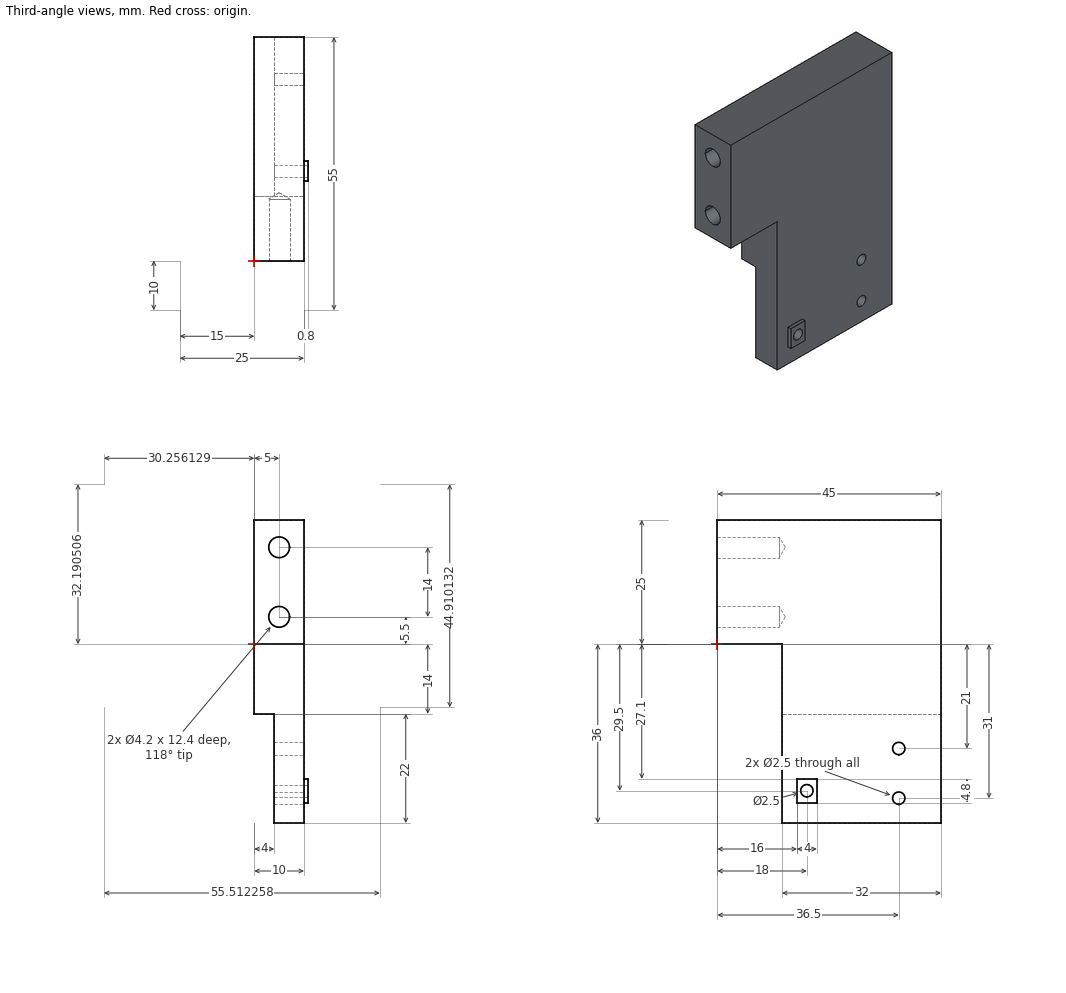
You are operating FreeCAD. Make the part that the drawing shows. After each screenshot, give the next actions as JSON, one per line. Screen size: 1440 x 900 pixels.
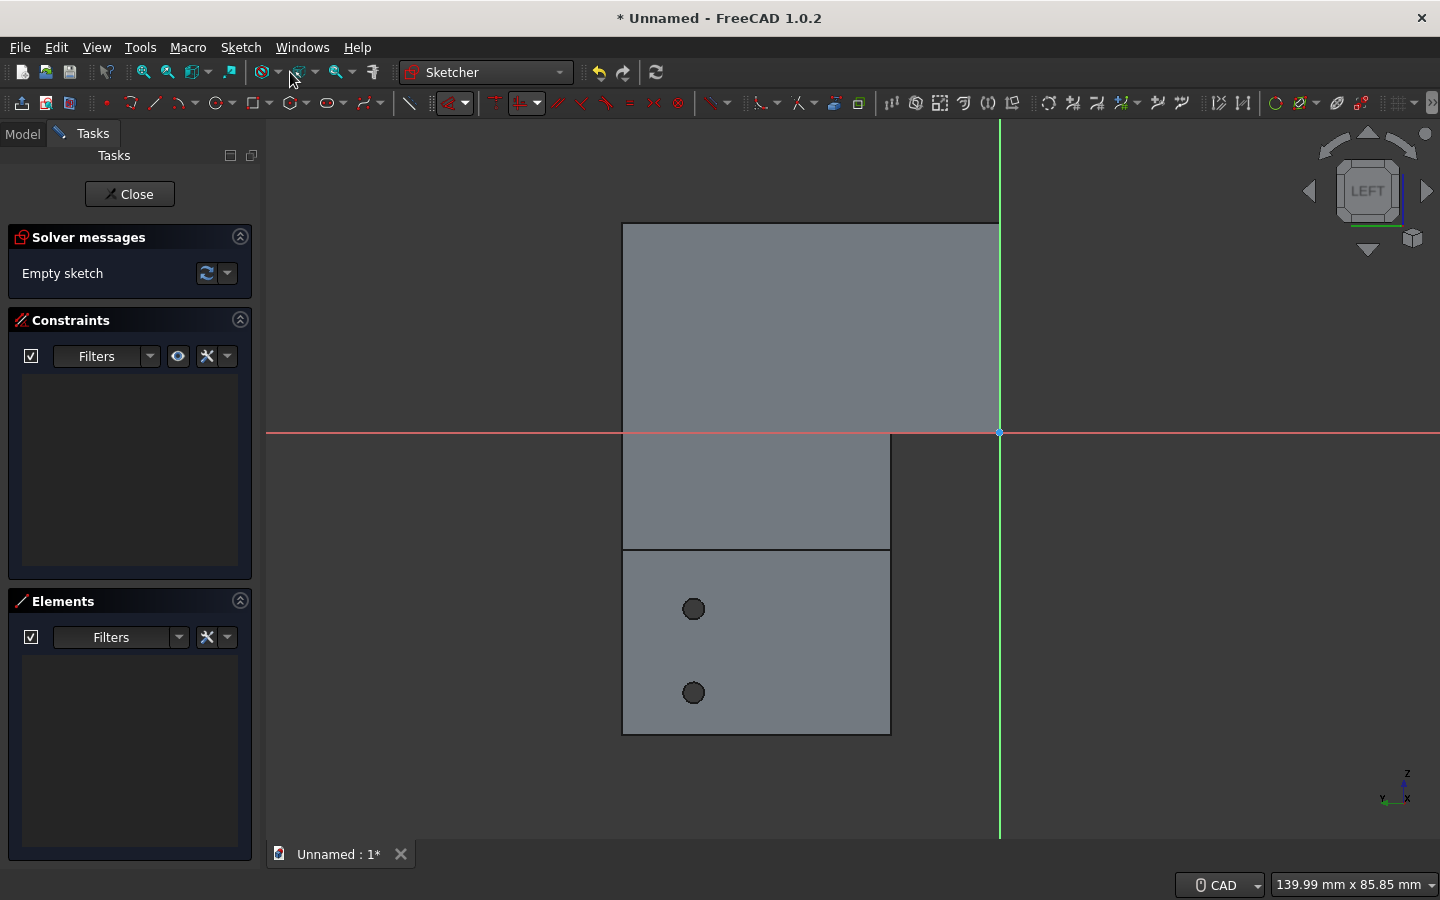
{"action": "scroll", "coordinate": [852, 691], "scroll_direction": "up", "scroll_amount": 15}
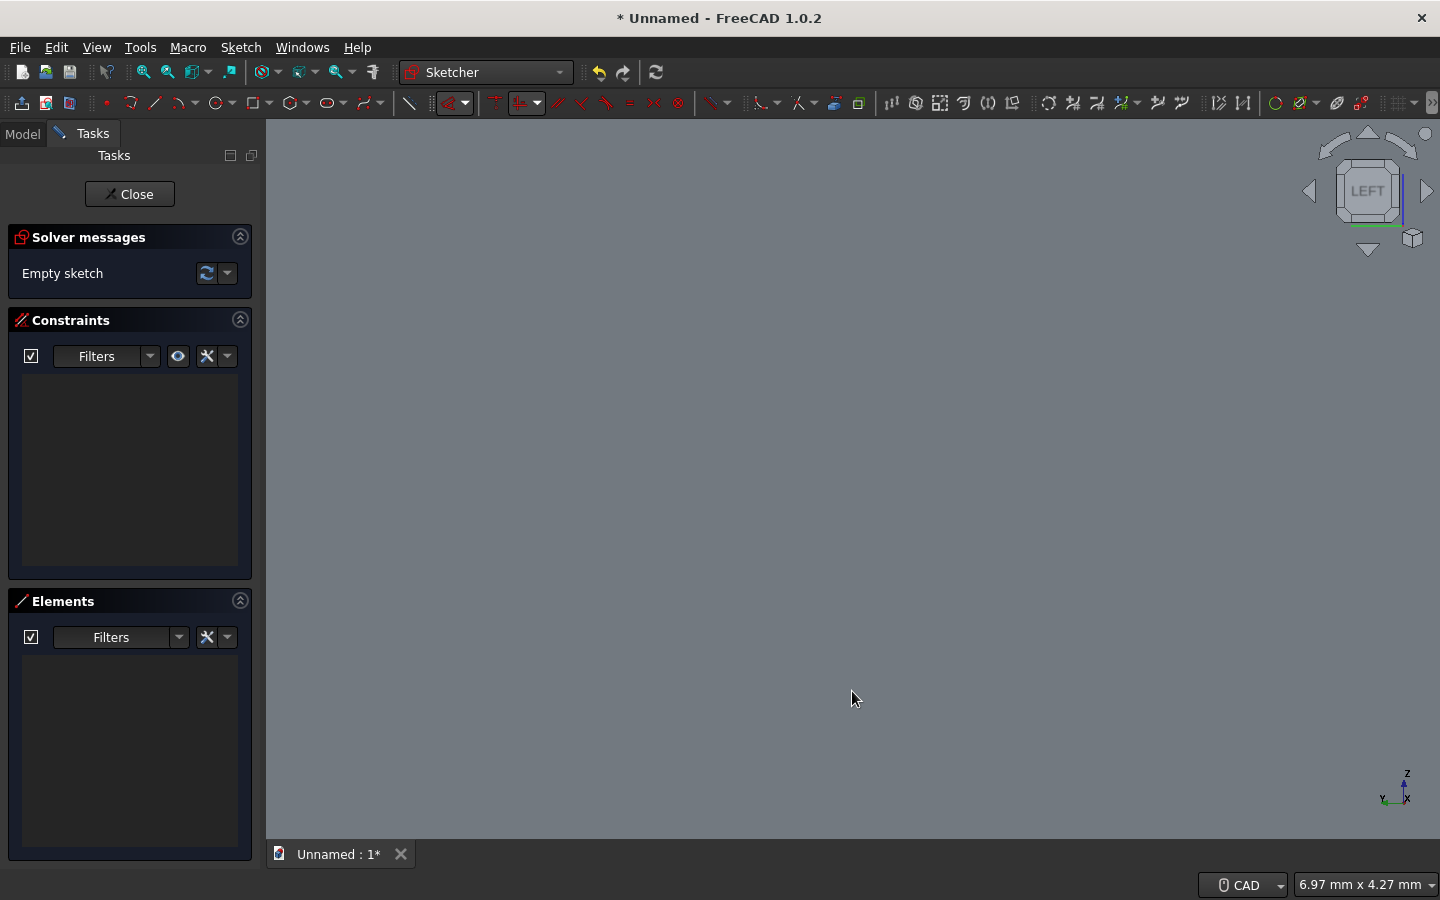
{"action": "left_click", "coordinate": [216, 104]}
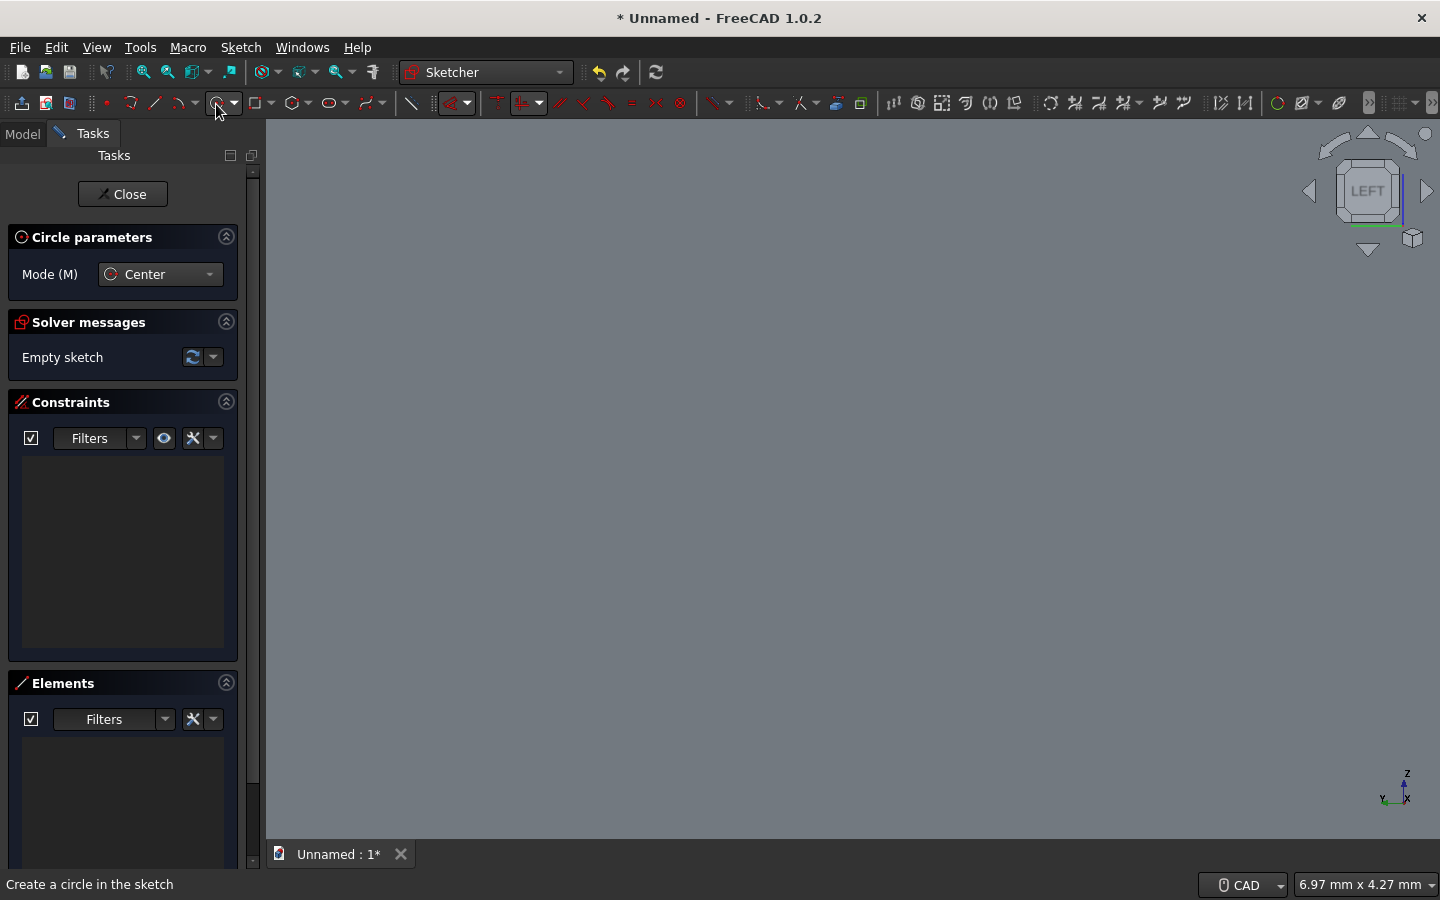
{"action": "left_click", "coordinate": [778, 460]}
{"action": "mouse_move", "coordinate": [927, 311]}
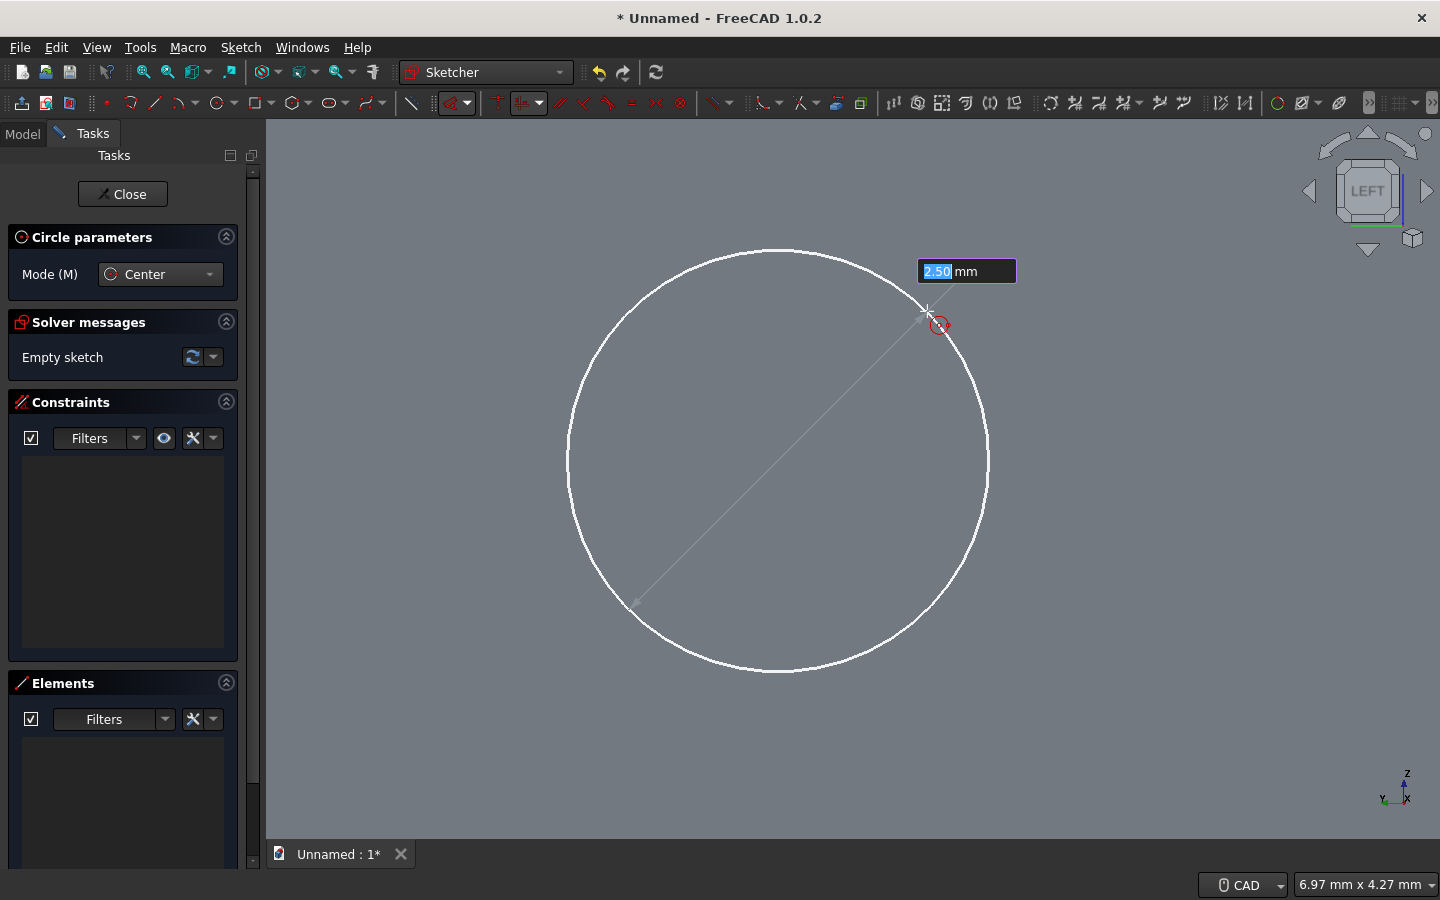
{"action": "type", "text": "2.5"}
{"action": "key", "text": "Return"}
{"action": "key", "text": "Escape"}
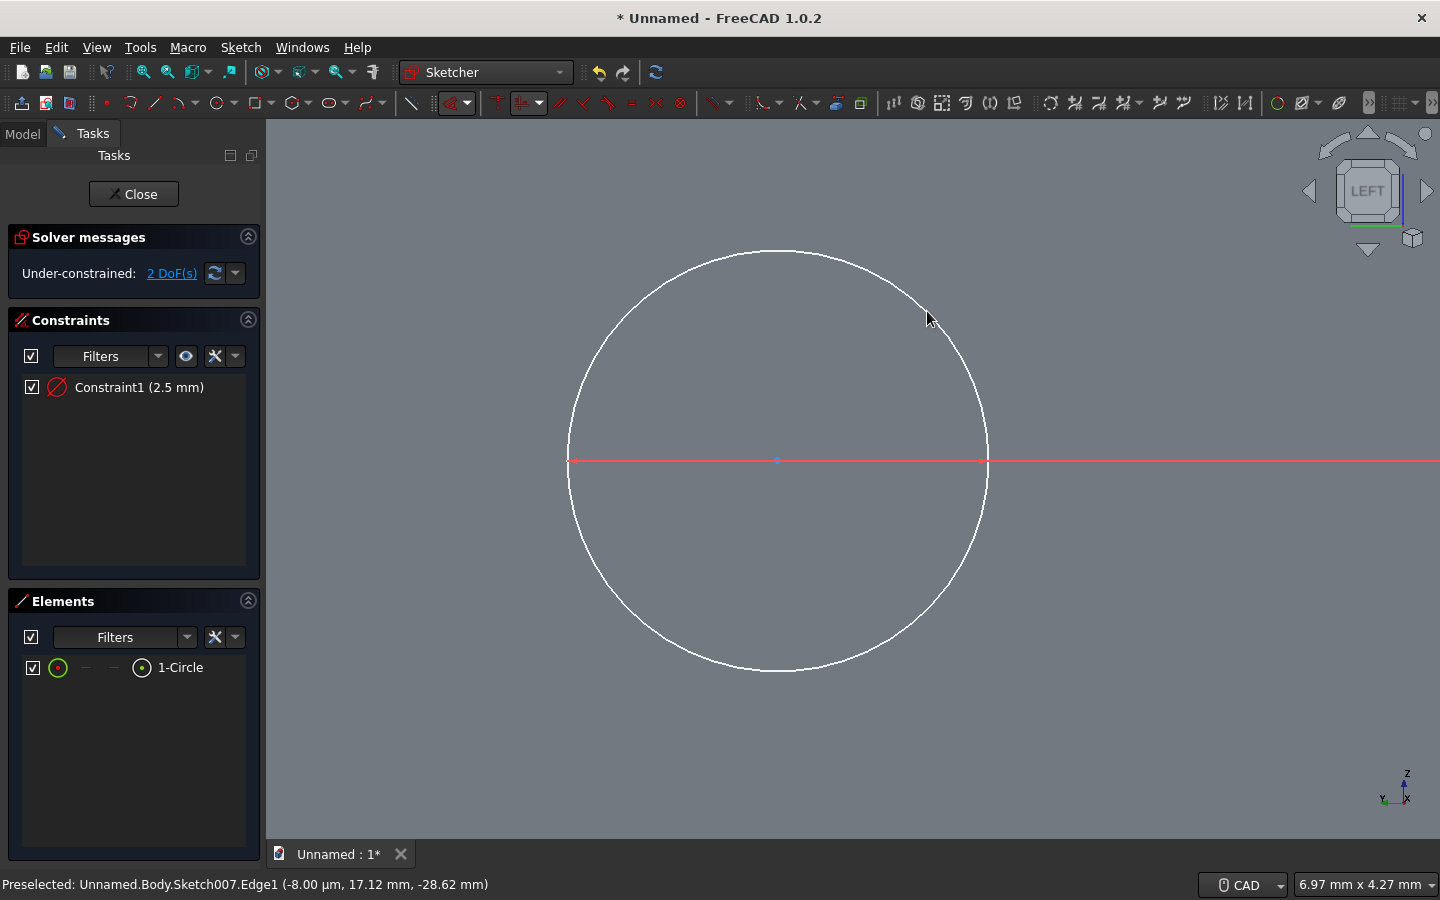
{"action": "left_click", "coordinate": [778, 461]}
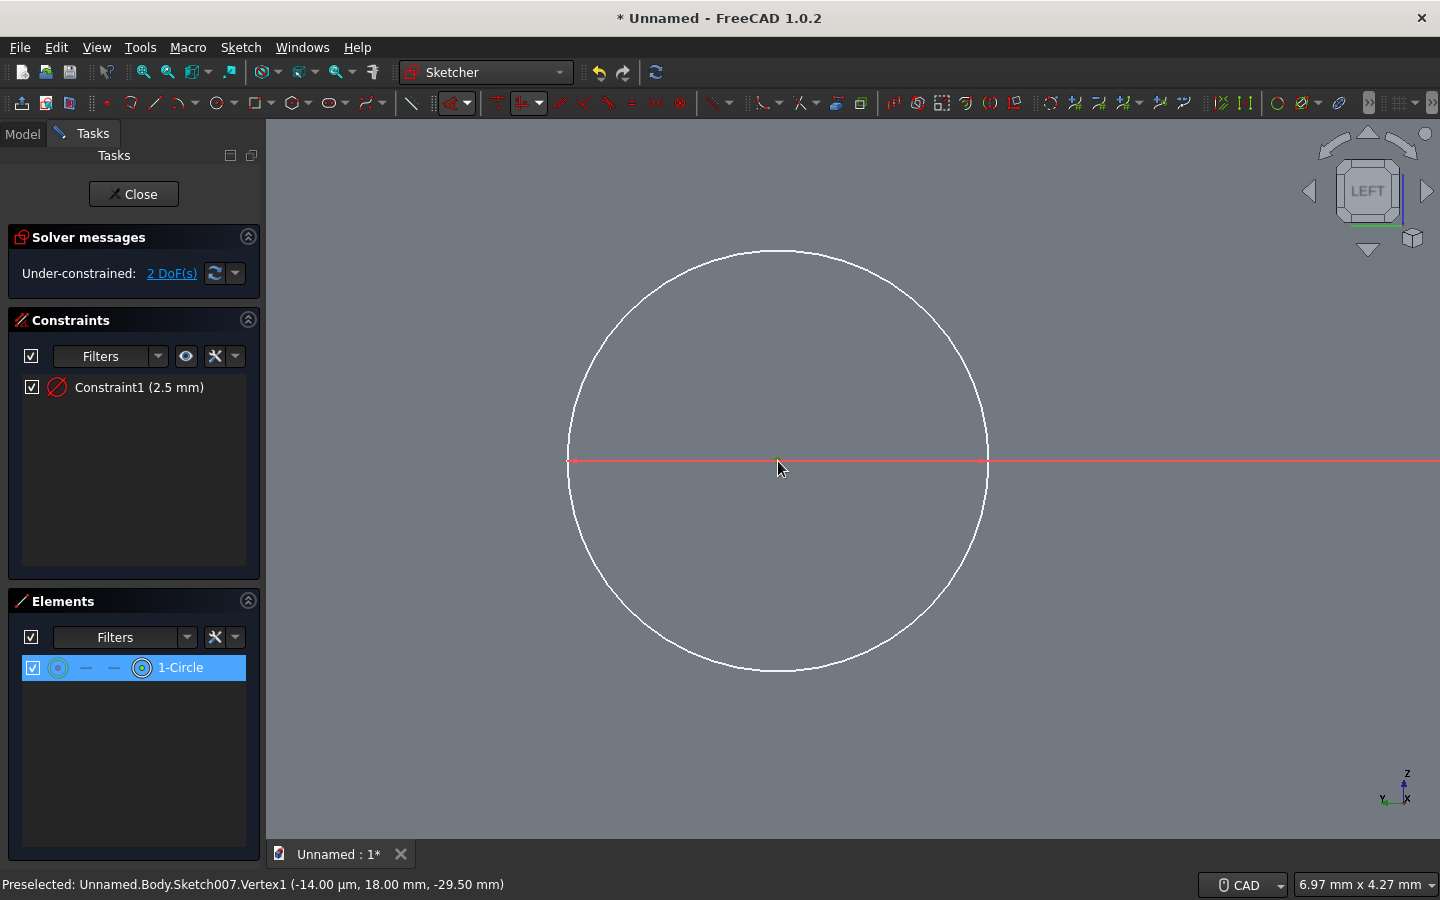
{"action": "key", "text": "l"}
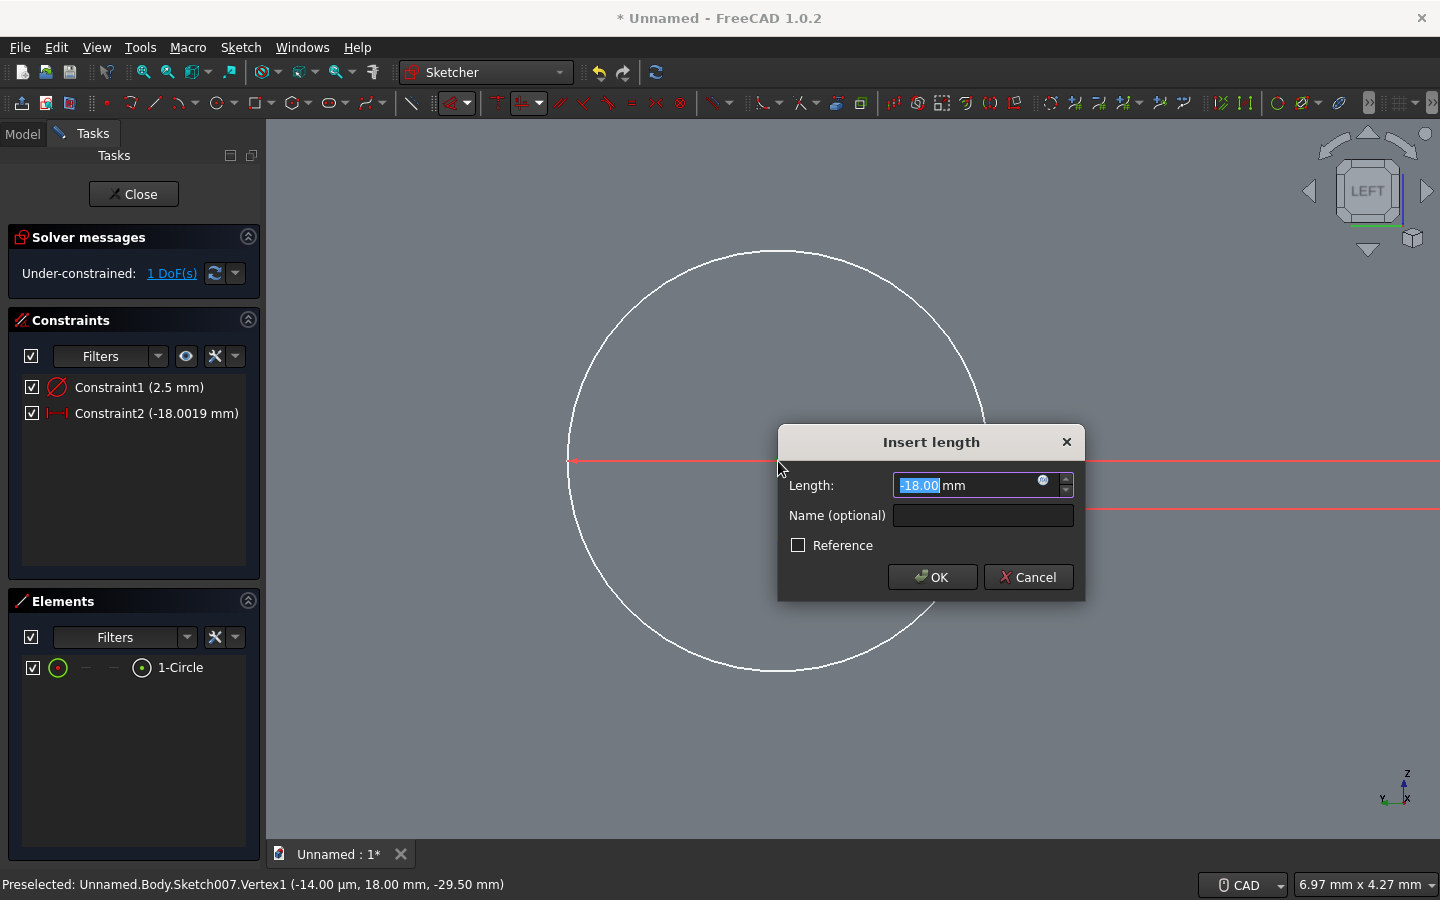
{"action": "type", "text": "-18"}
{"action": "key", "text": "Return"}